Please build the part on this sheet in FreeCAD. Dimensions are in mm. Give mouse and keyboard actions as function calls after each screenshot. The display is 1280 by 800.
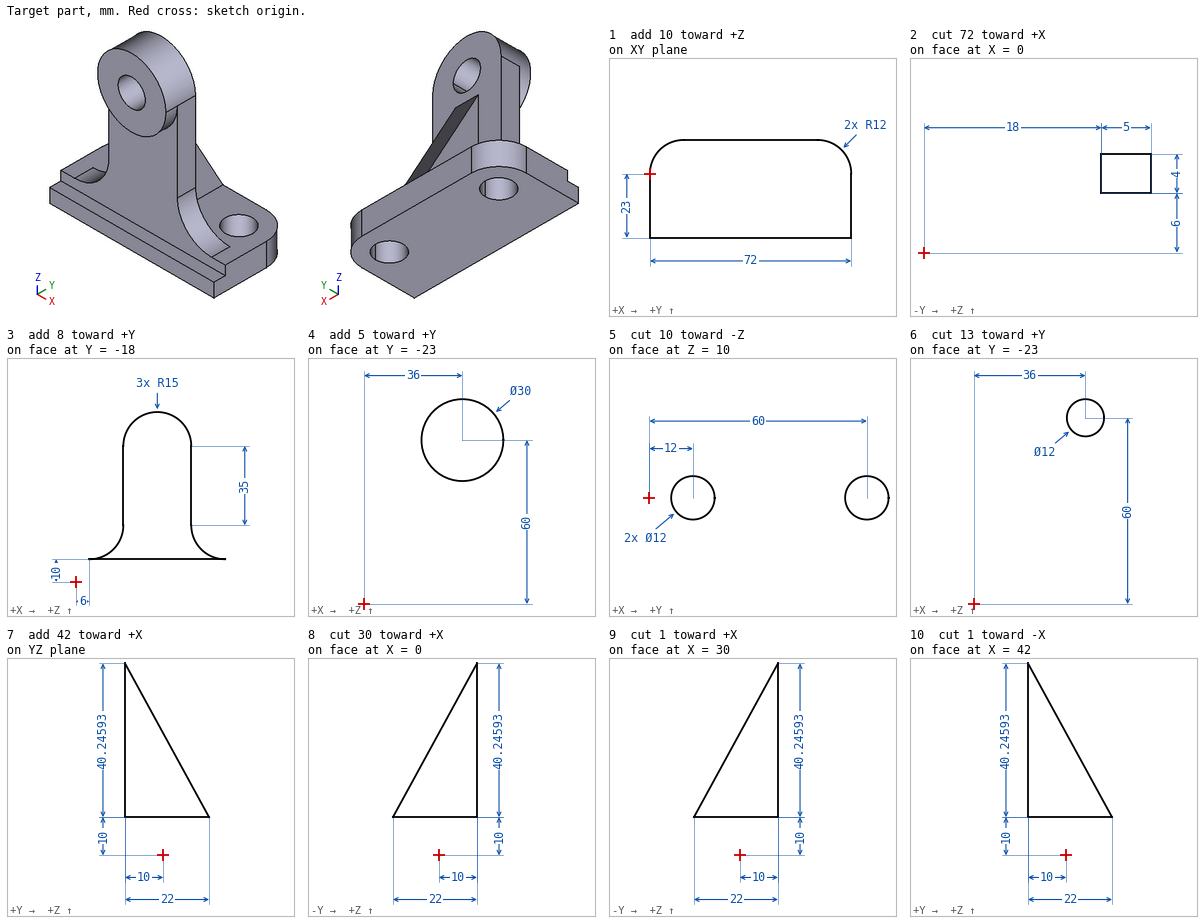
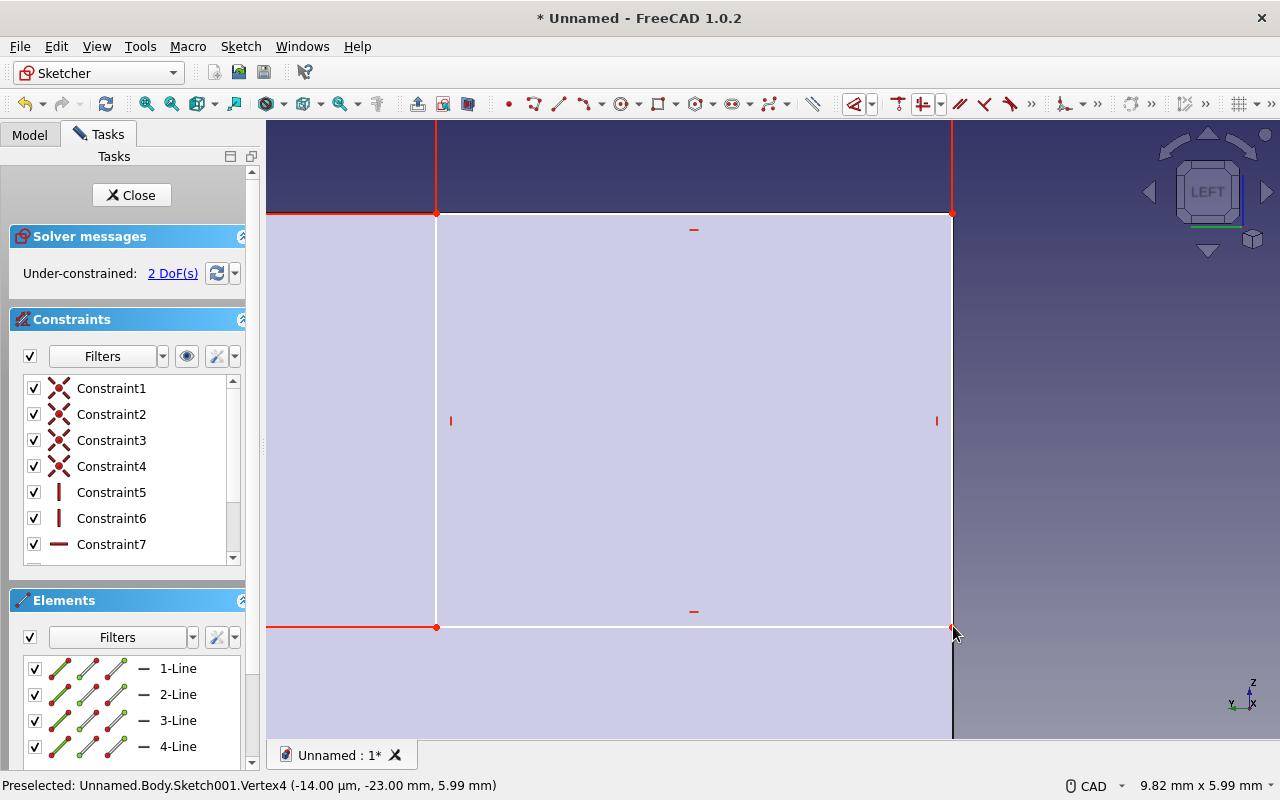
click(436, 627)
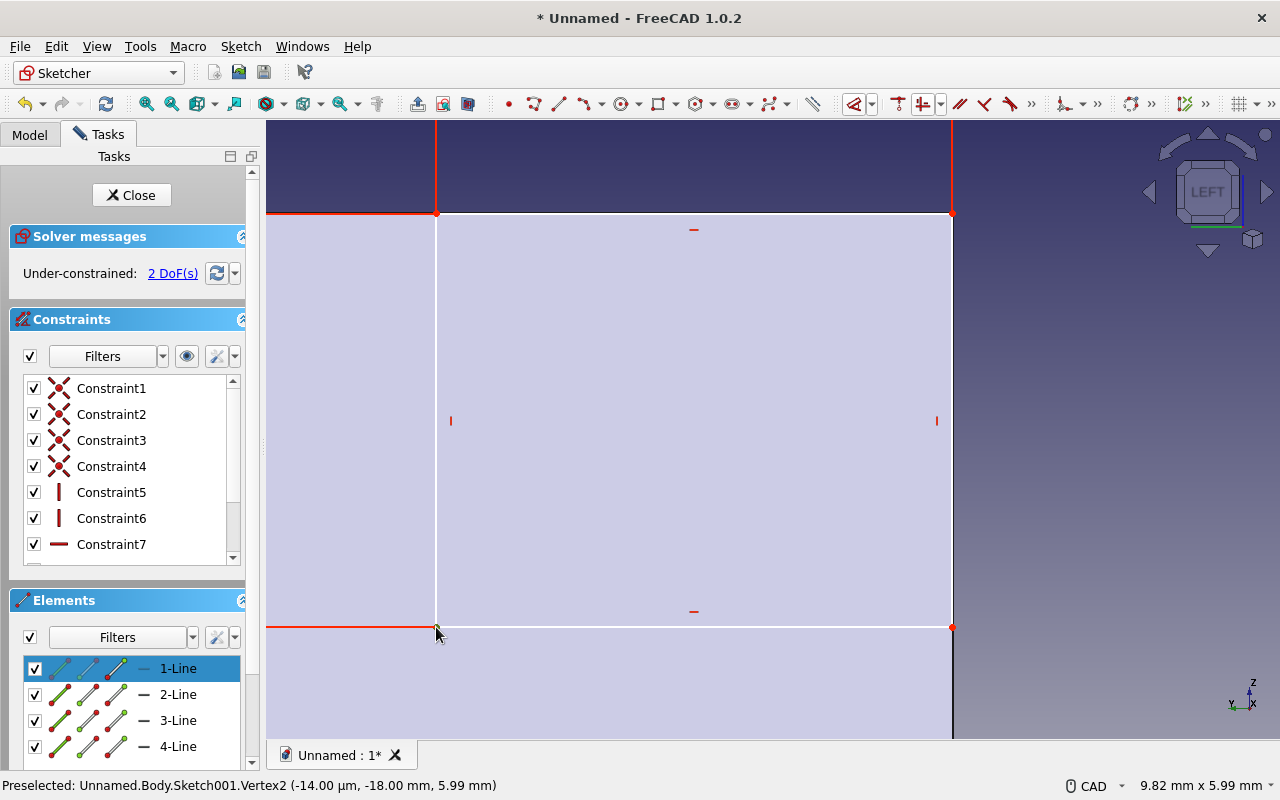
click(872, 104)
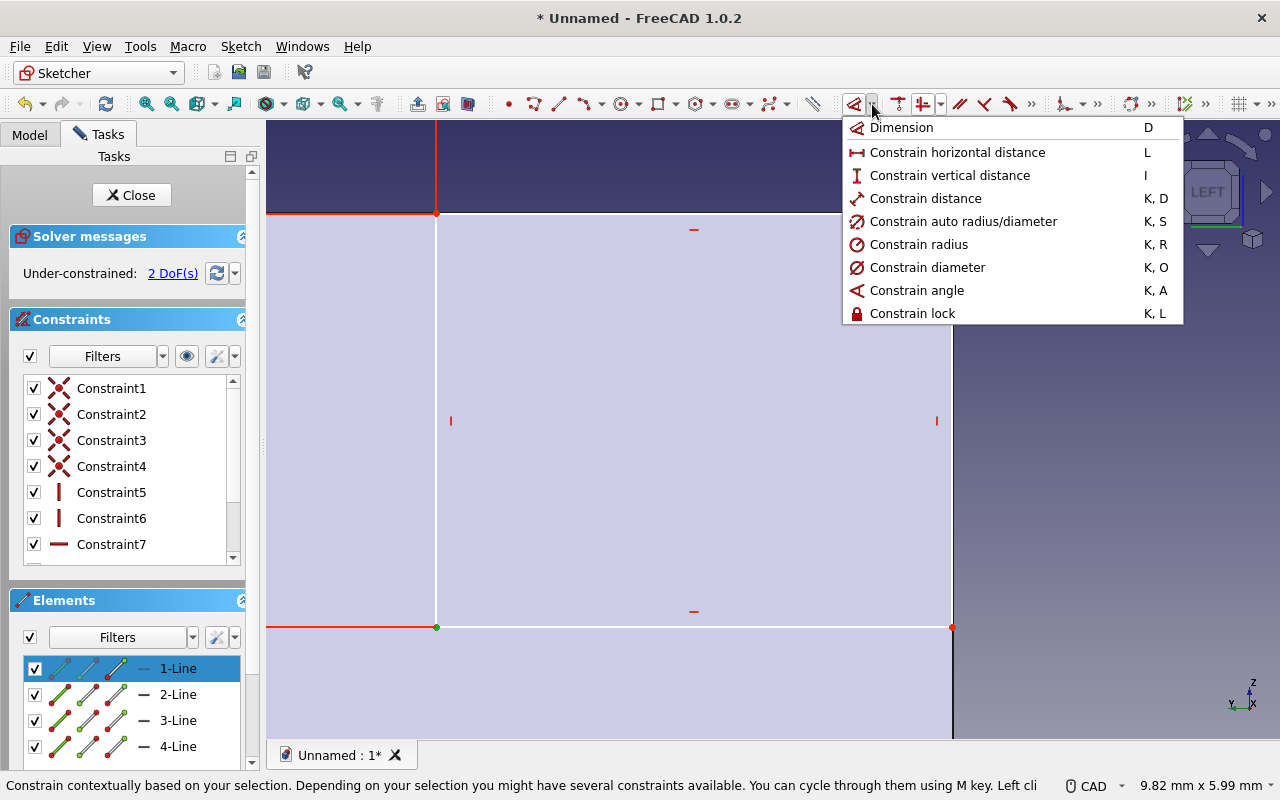
click(1013, 176)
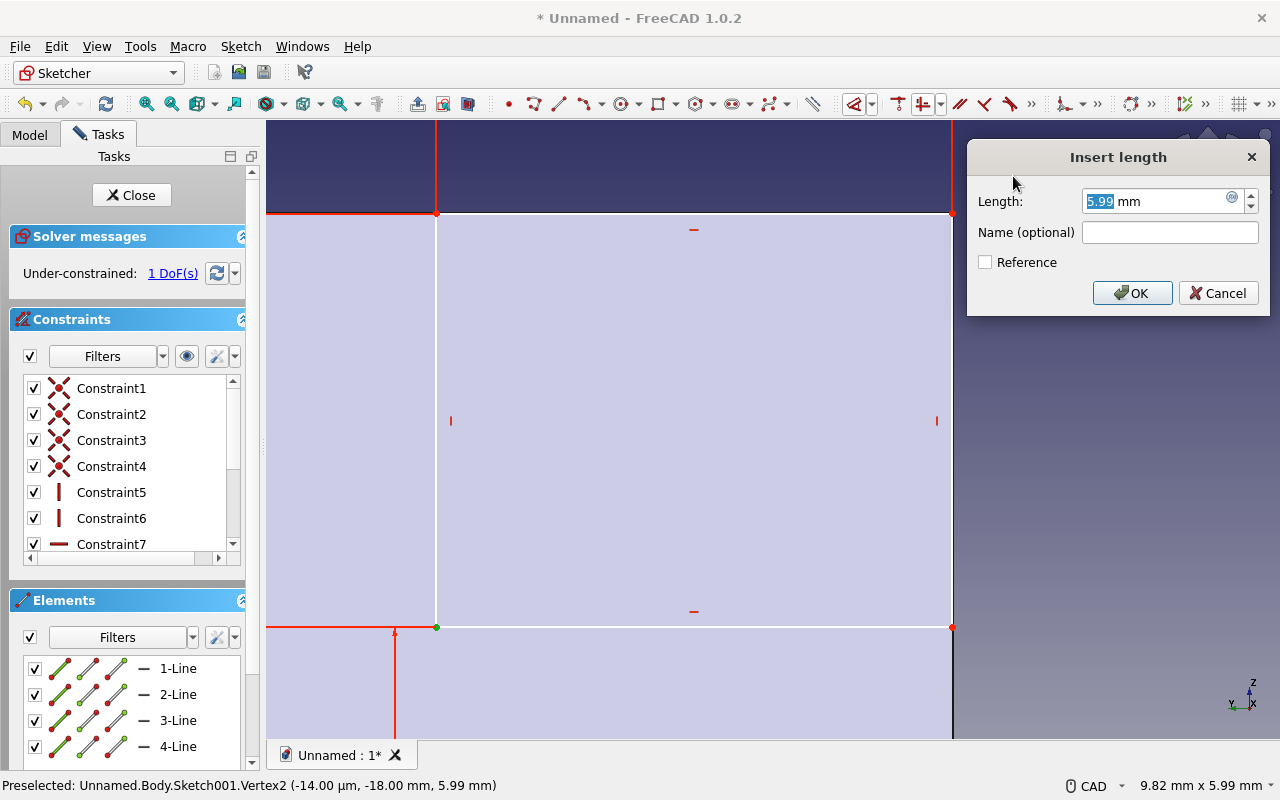
text(6)
key(Return)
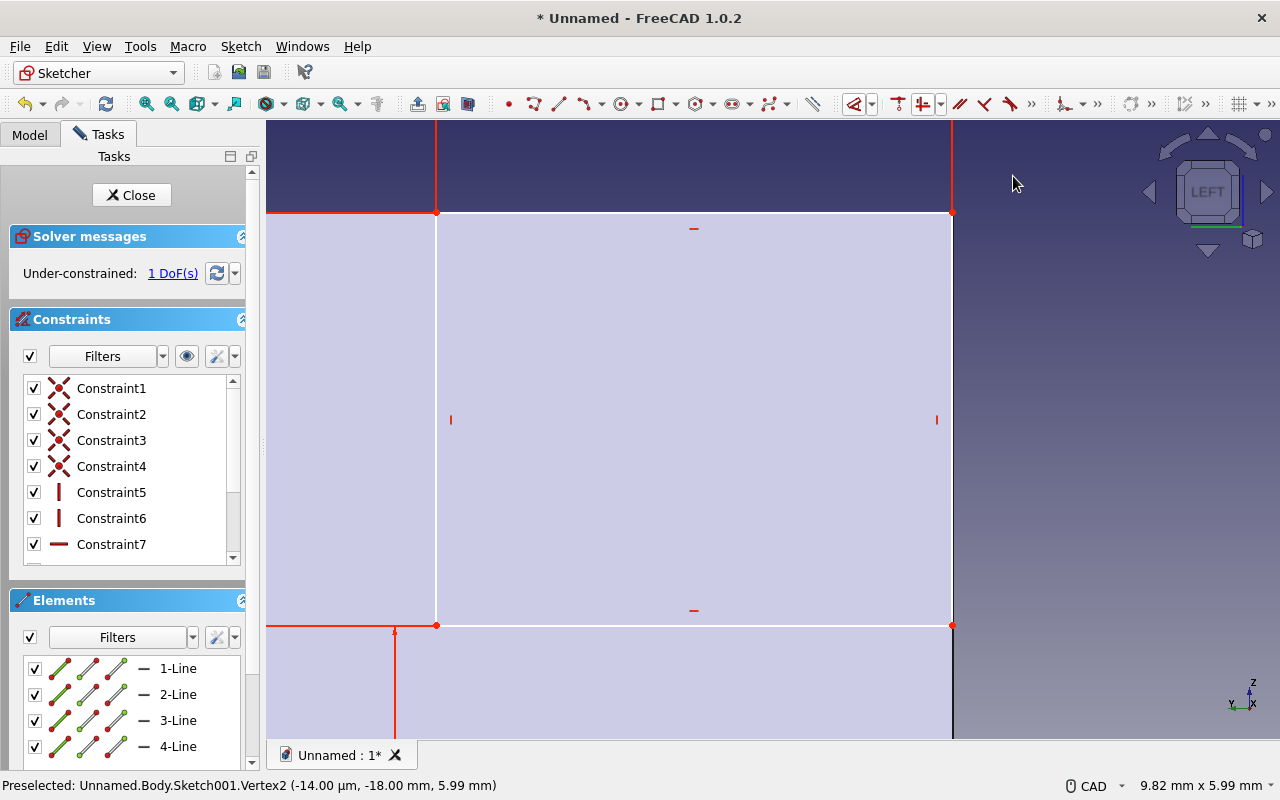
click(436, 213)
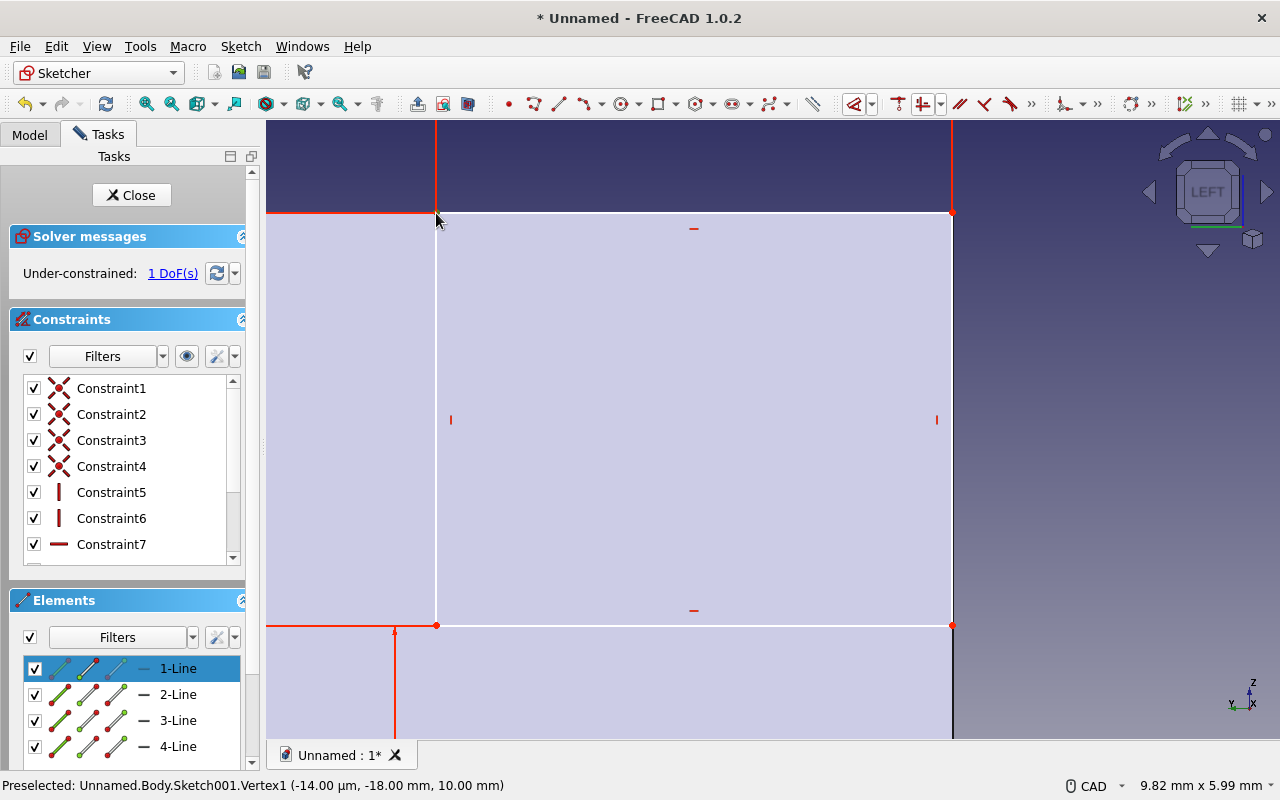
click(872, 104)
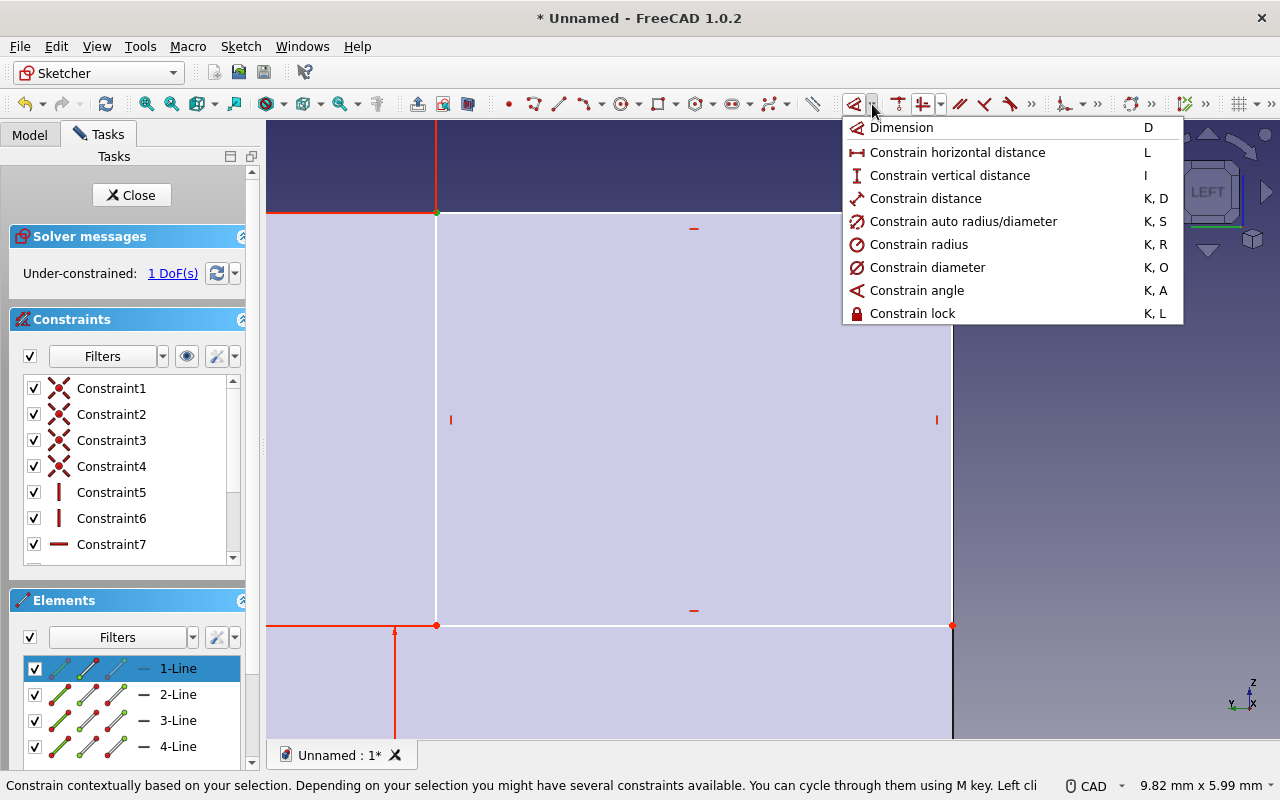
click(1013, 152)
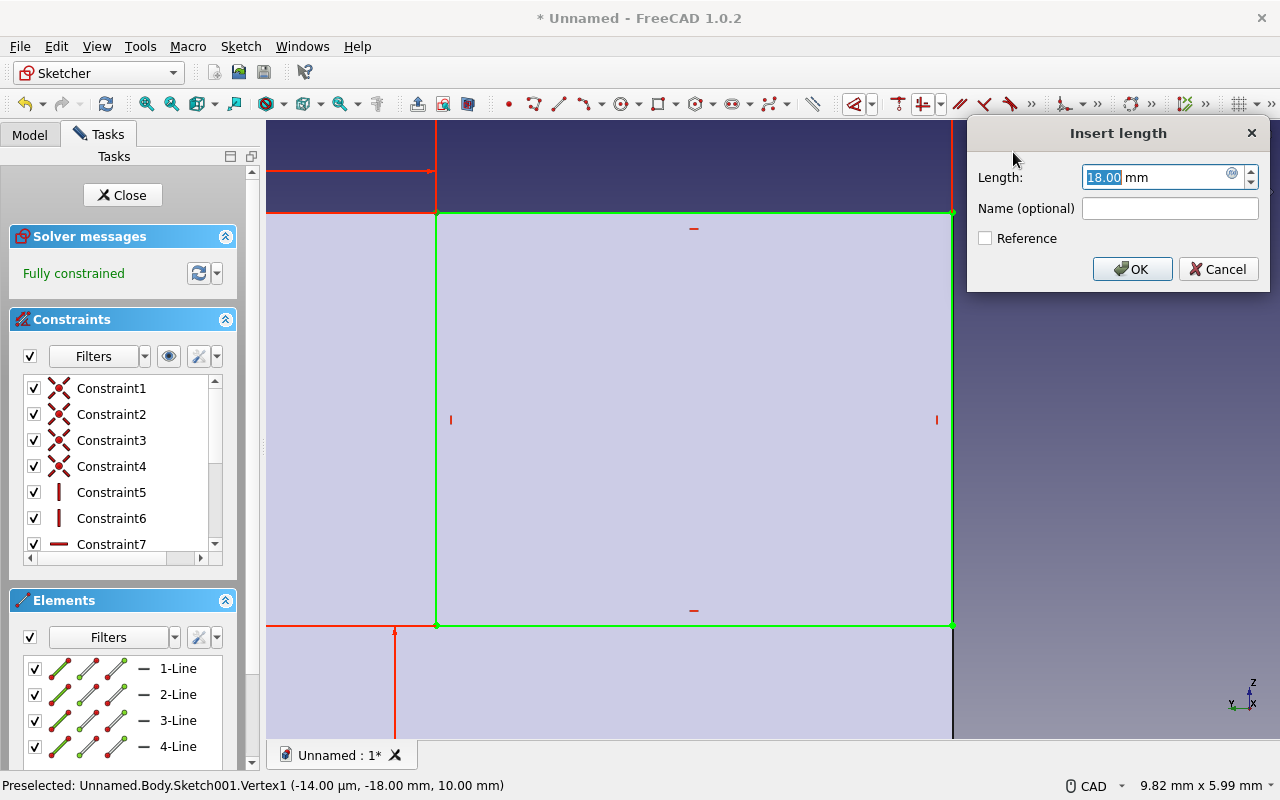
text(18)
key(Return)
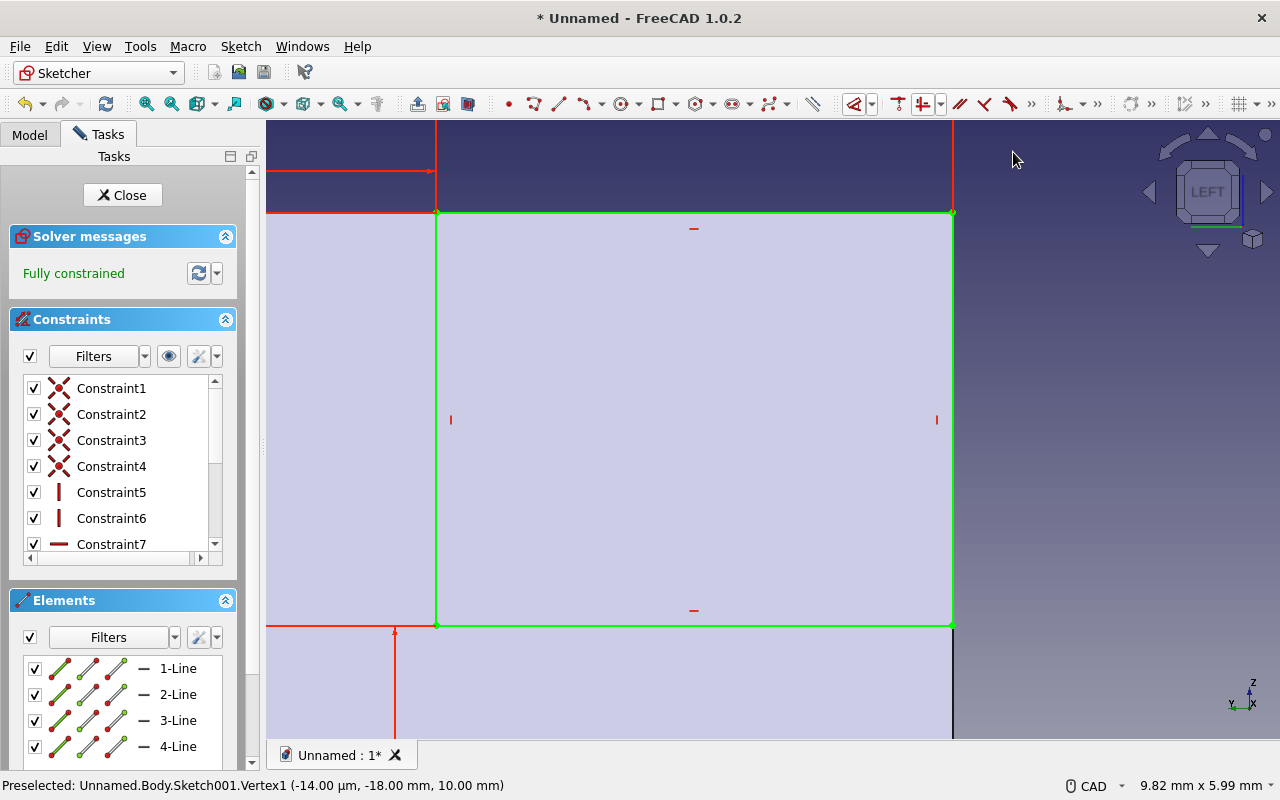
click(123, 195)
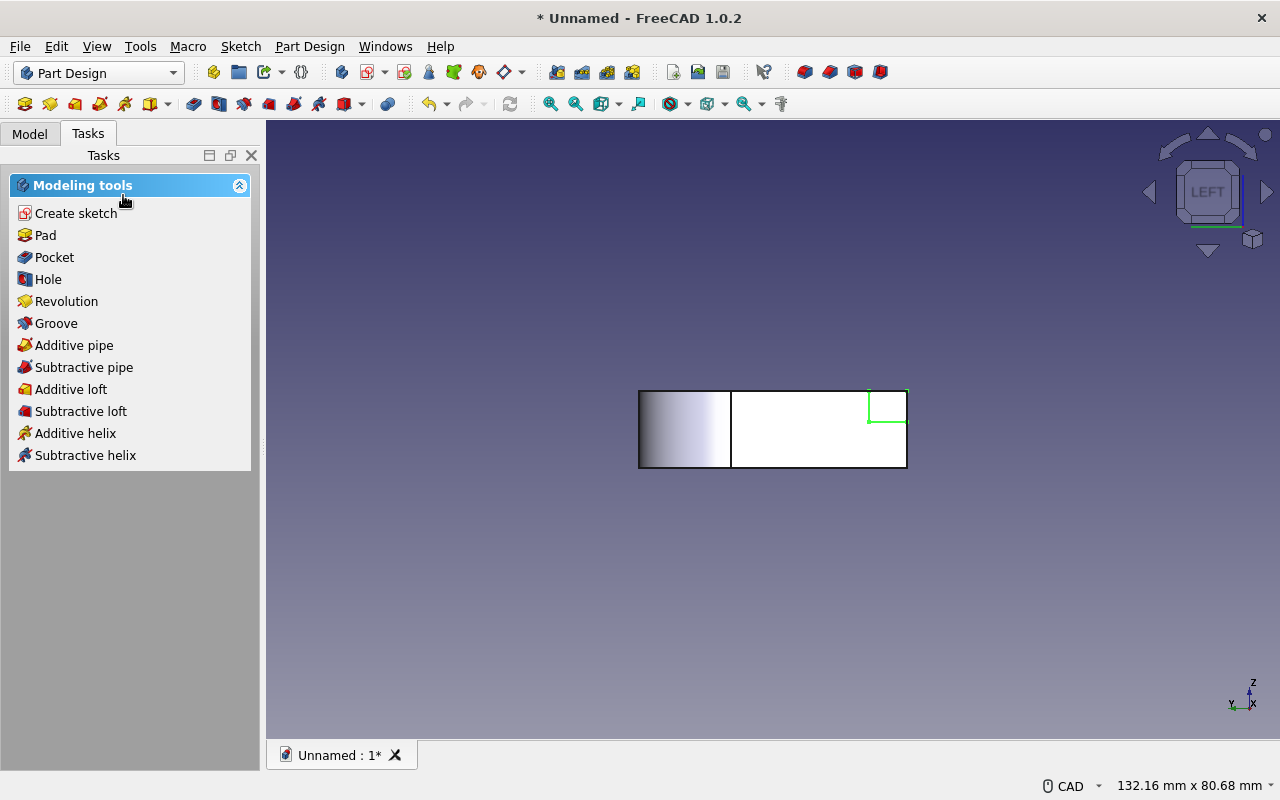
click(194, 104)